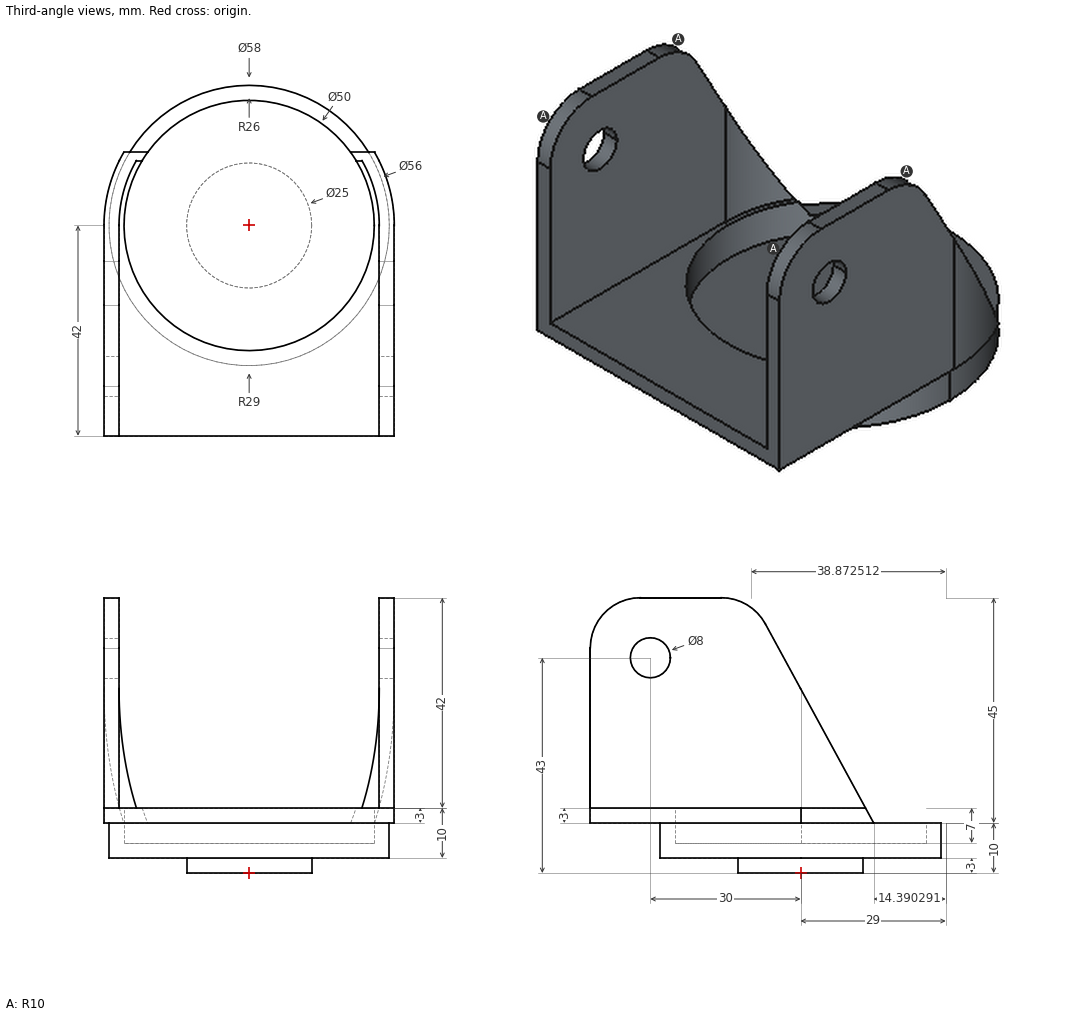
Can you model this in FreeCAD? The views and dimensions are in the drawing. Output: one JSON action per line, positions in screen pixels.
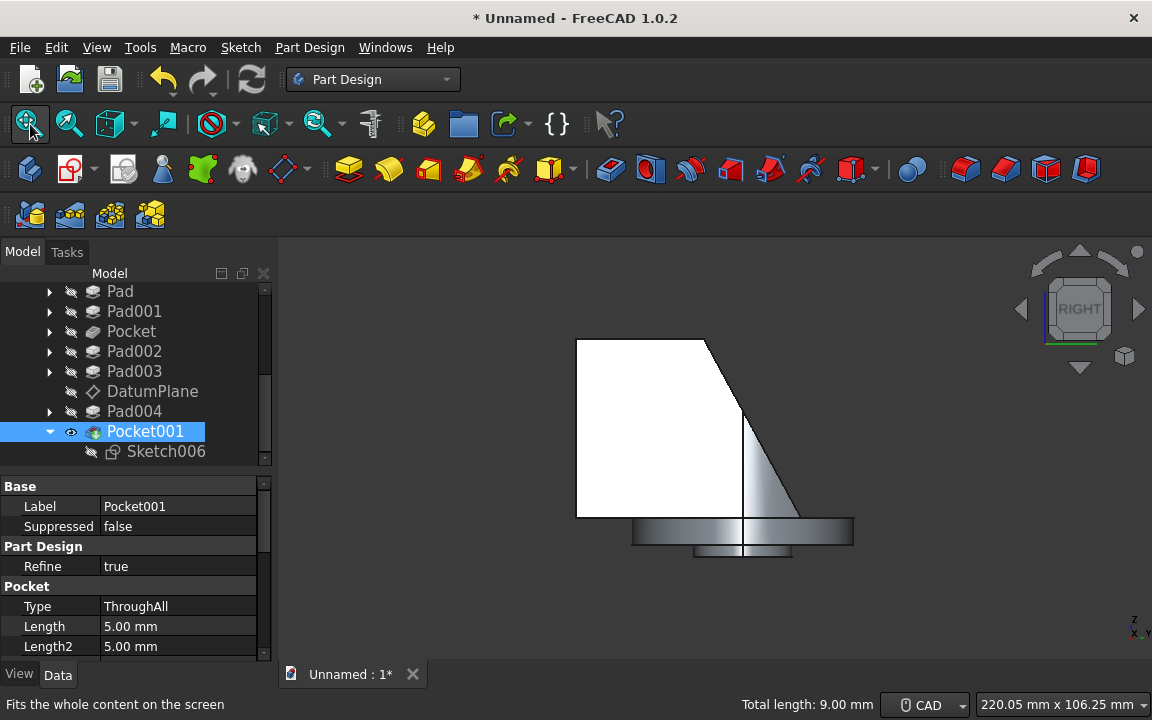
{"action": "scroll", "coordinate": [704, 338], "scroll_direction": "up", "scroll_amount": 7}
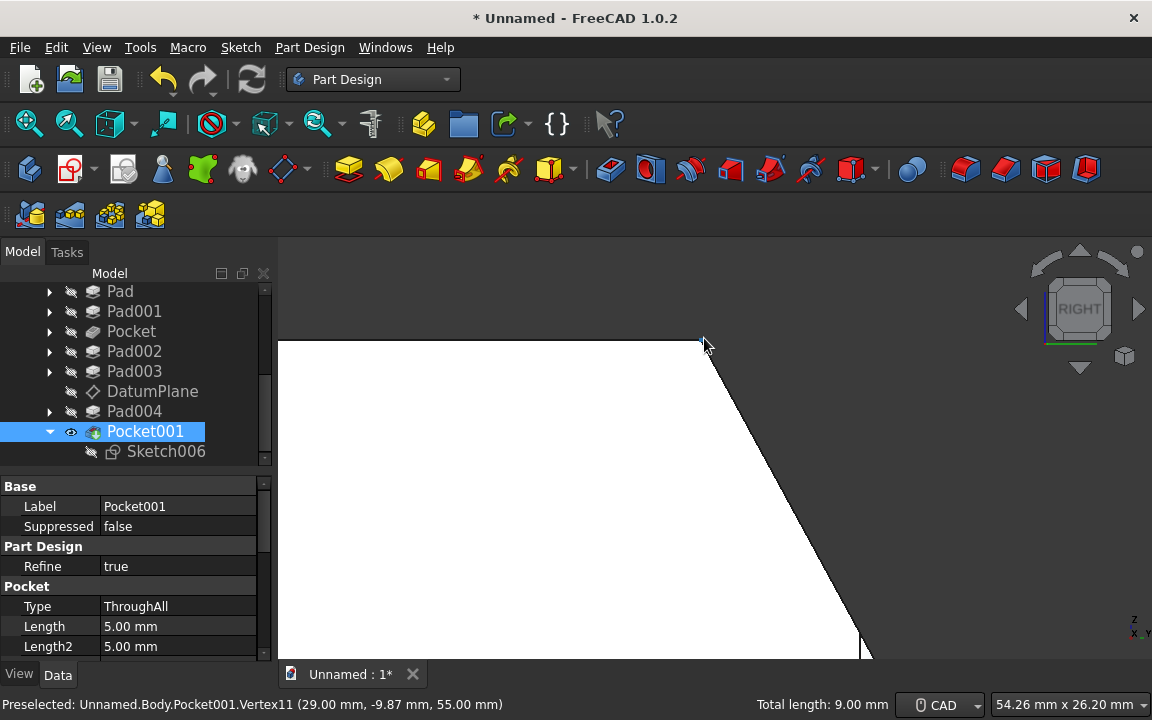
{"action": "left_click", "coordinate": [30, 124]}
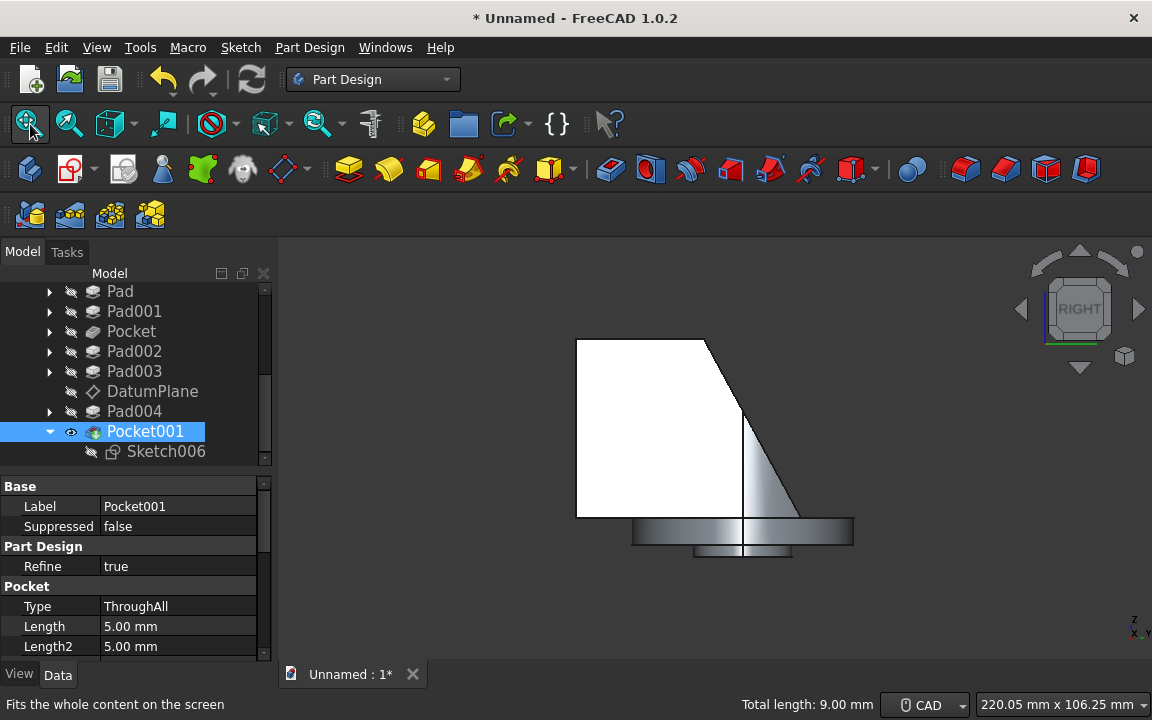
{"action": "key", "text": "5"}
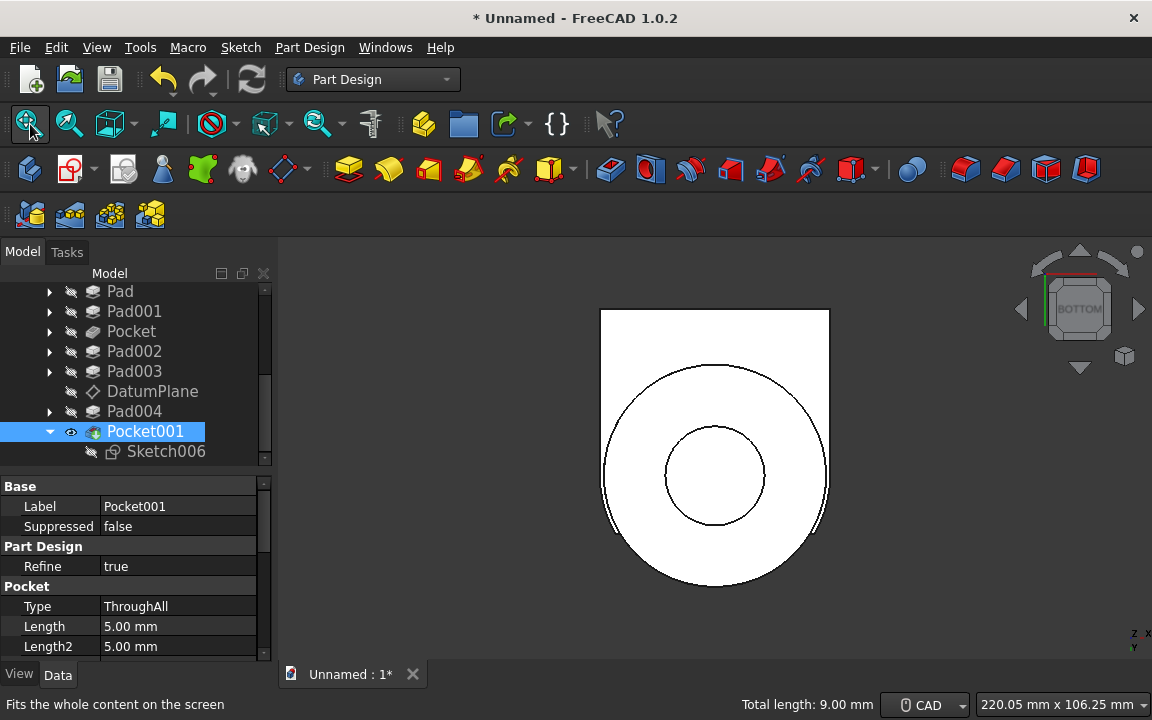
{"action": "scroll", "coordinate": [606, 436], "scroll_direction": "up", "scroll_amount": 7}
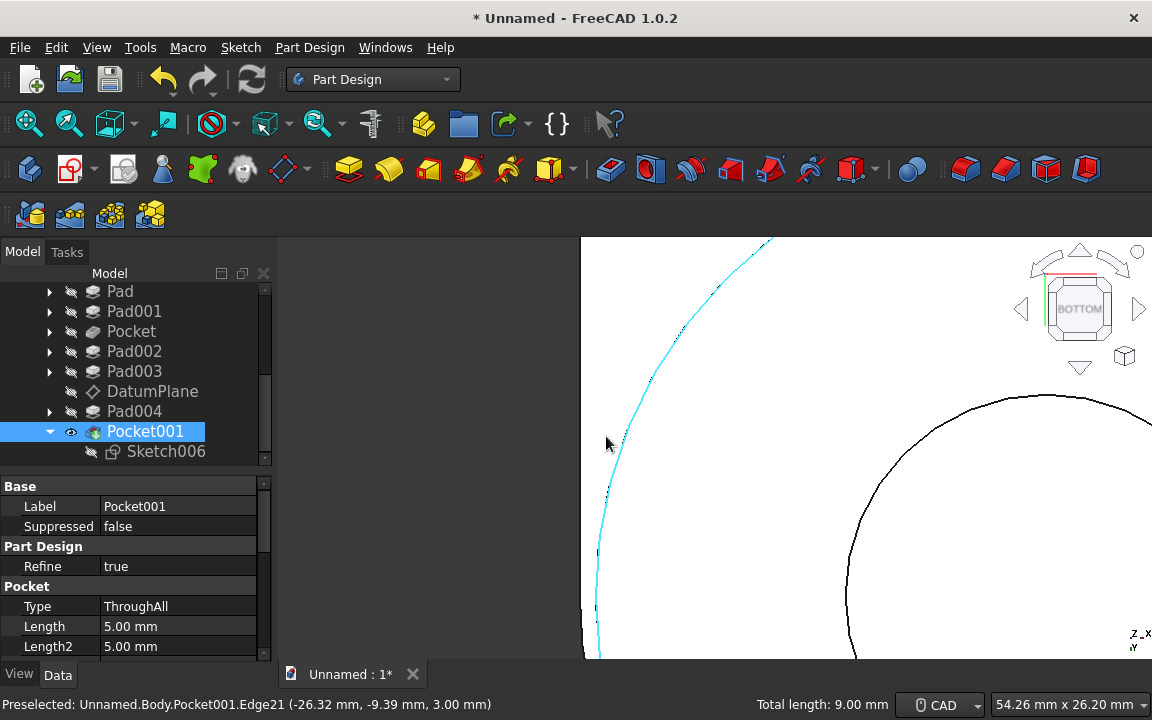
{"action": "left_click", "coordinate": [30, 124]}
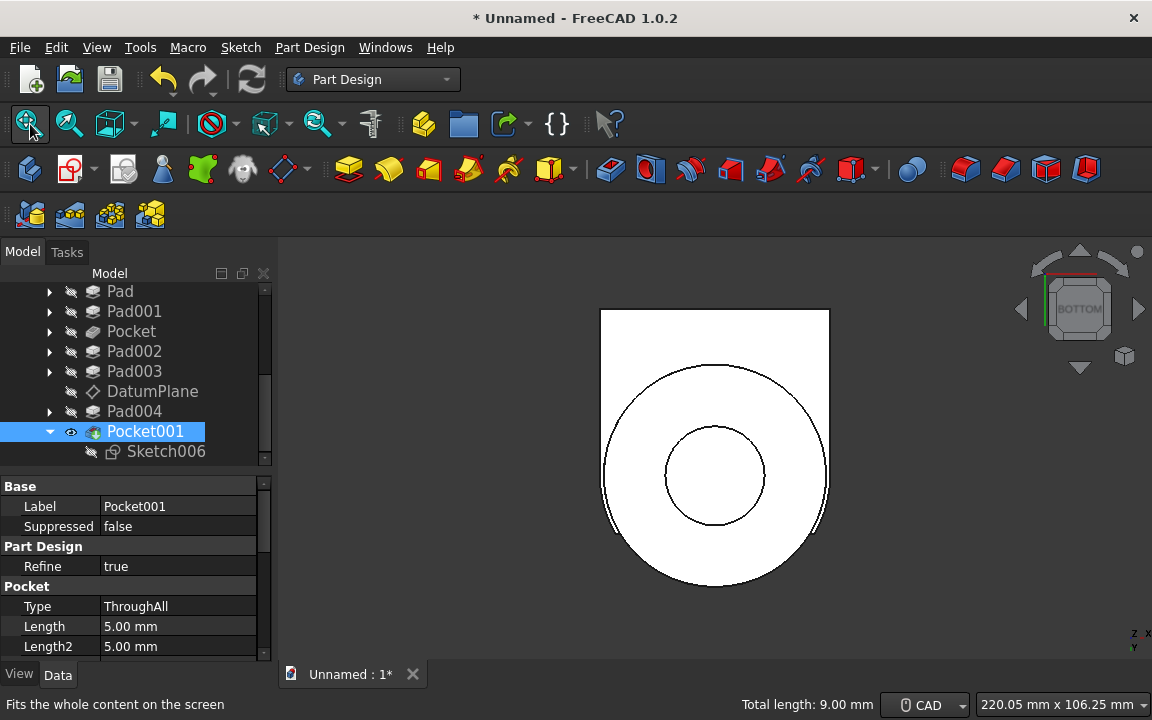
{"action": "key", "text": "4"}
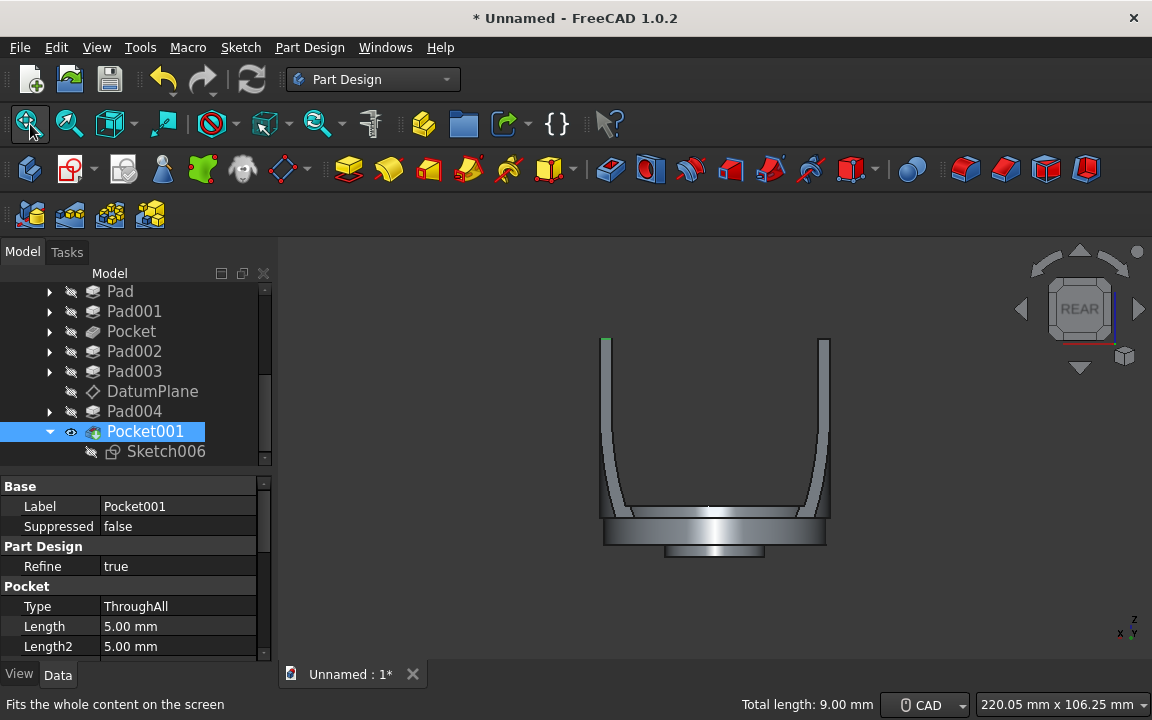
{"action": "scroll", "coordinate": [824, 338], "scroll_direction": "up", "scroll_amount": 7}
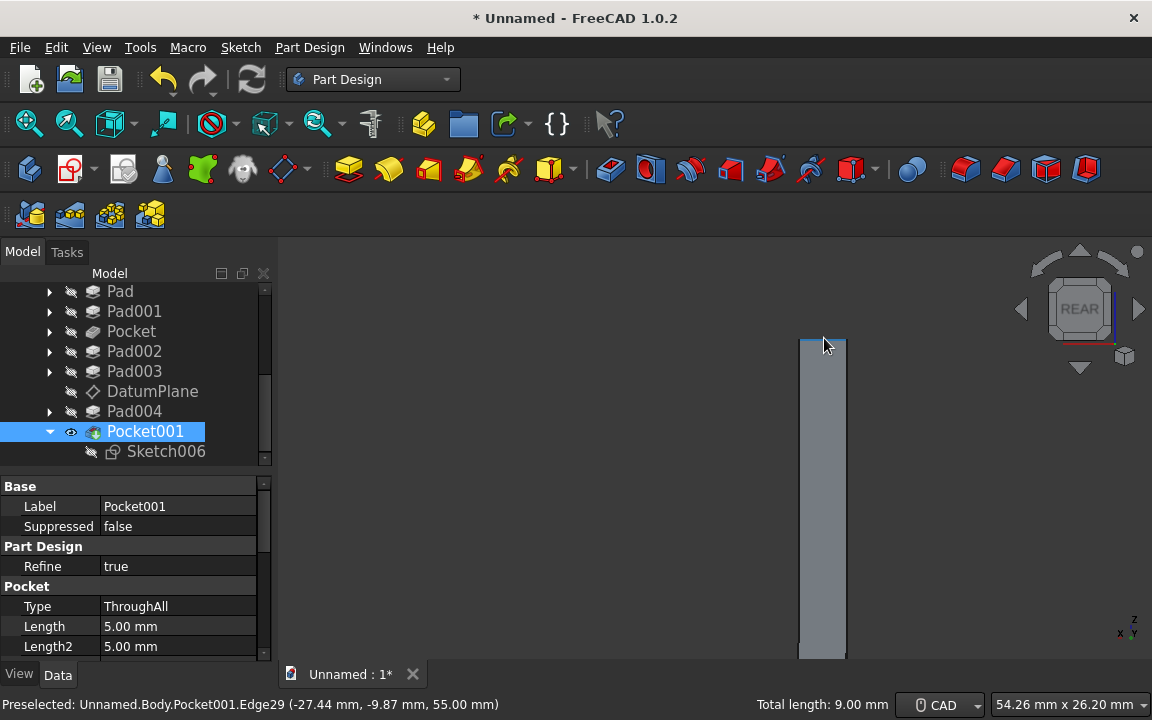
{"action": "left_click", "coordinate": [30, 124]}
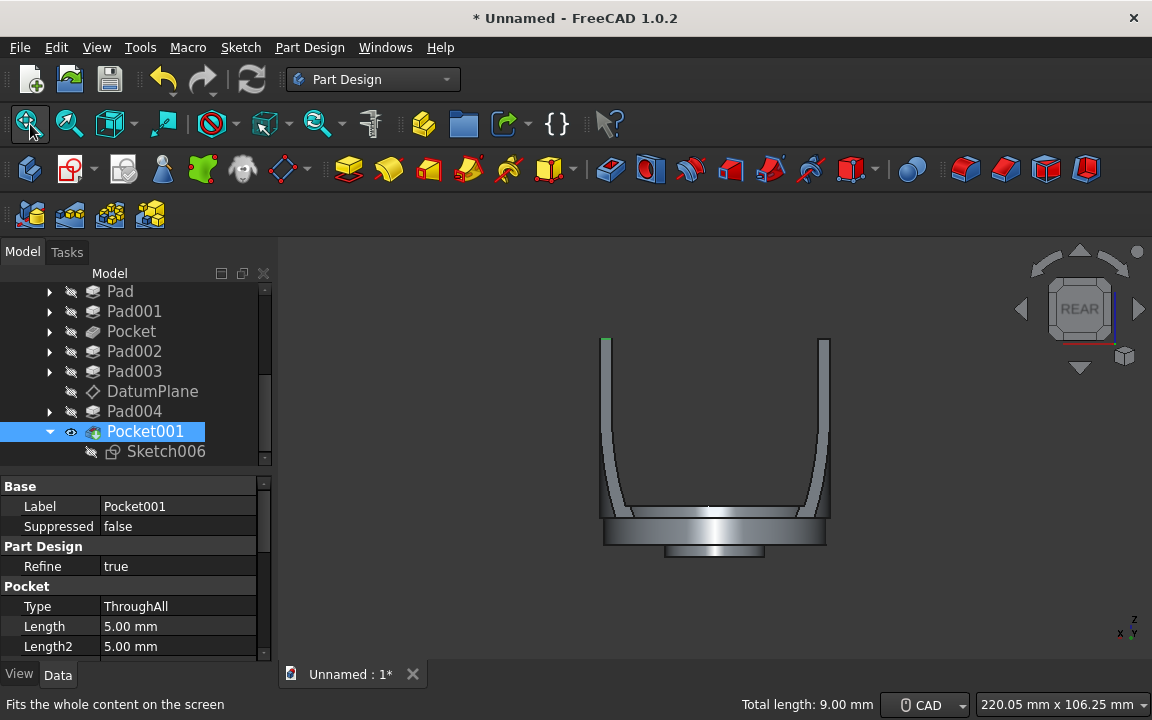
{"action": "key", "text": "6"}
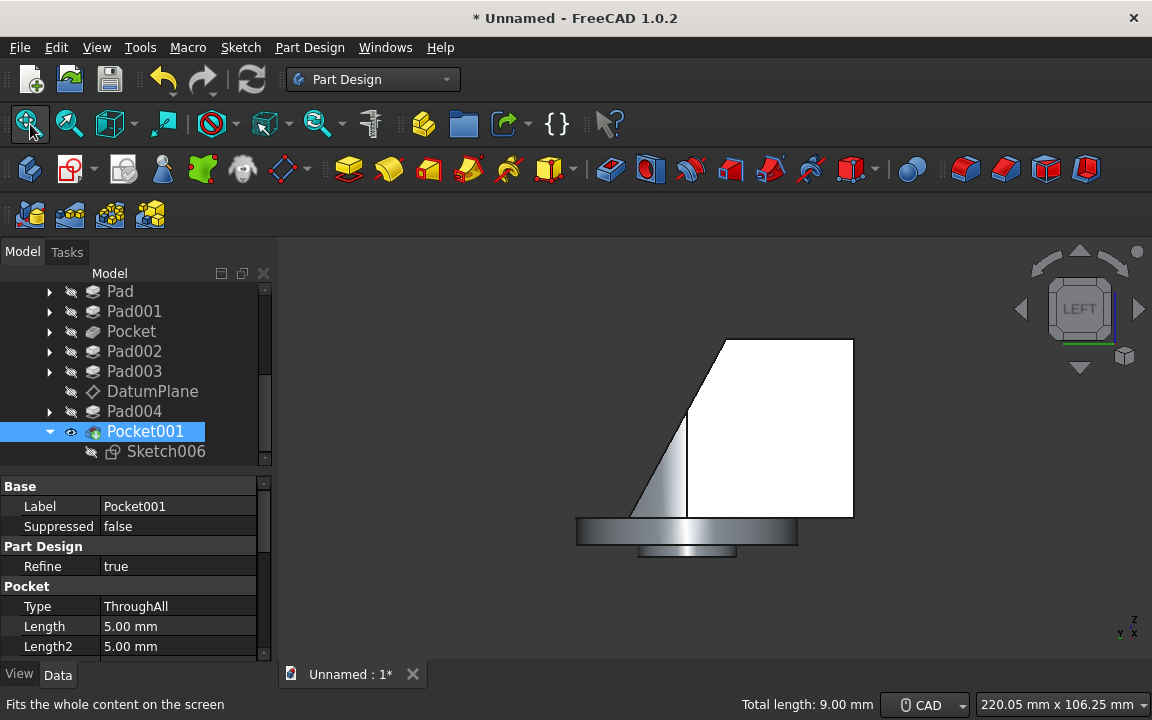
{"action": "scroll", "coordinate": [726, 338], "scroll_direction": "up", "scroll_amount": 7}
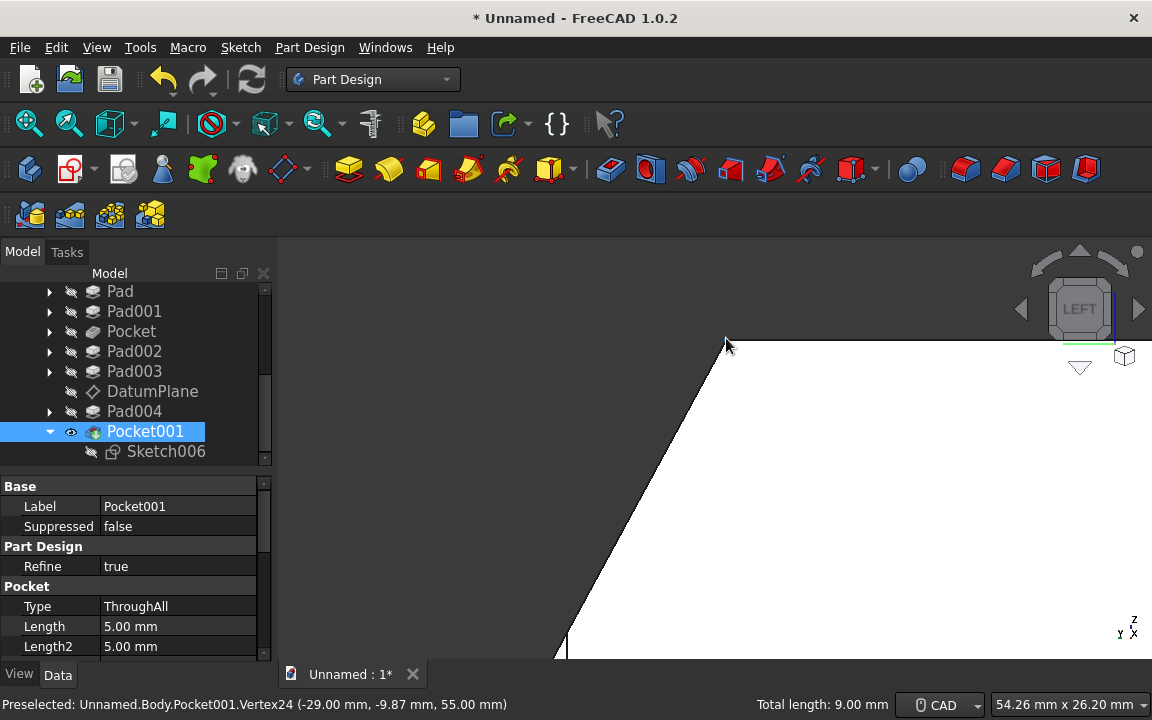
{"action": "left_click", "coordinate": [30, 124]}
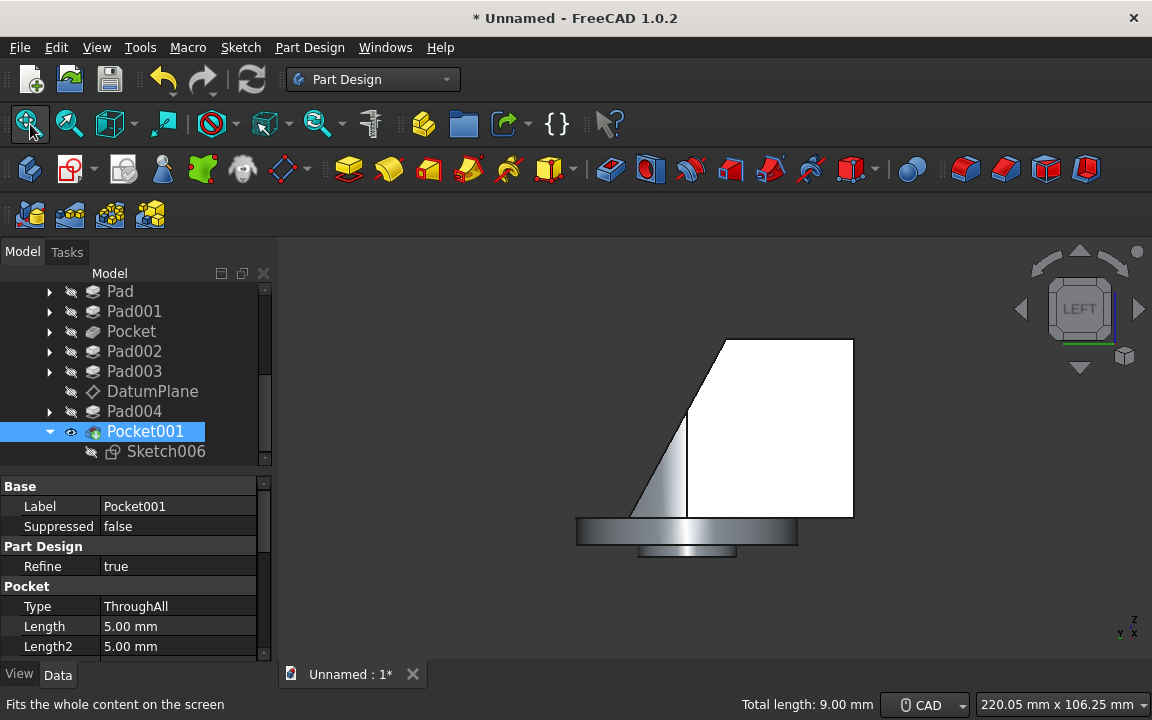
{"action": "key", "text": "v 3"}